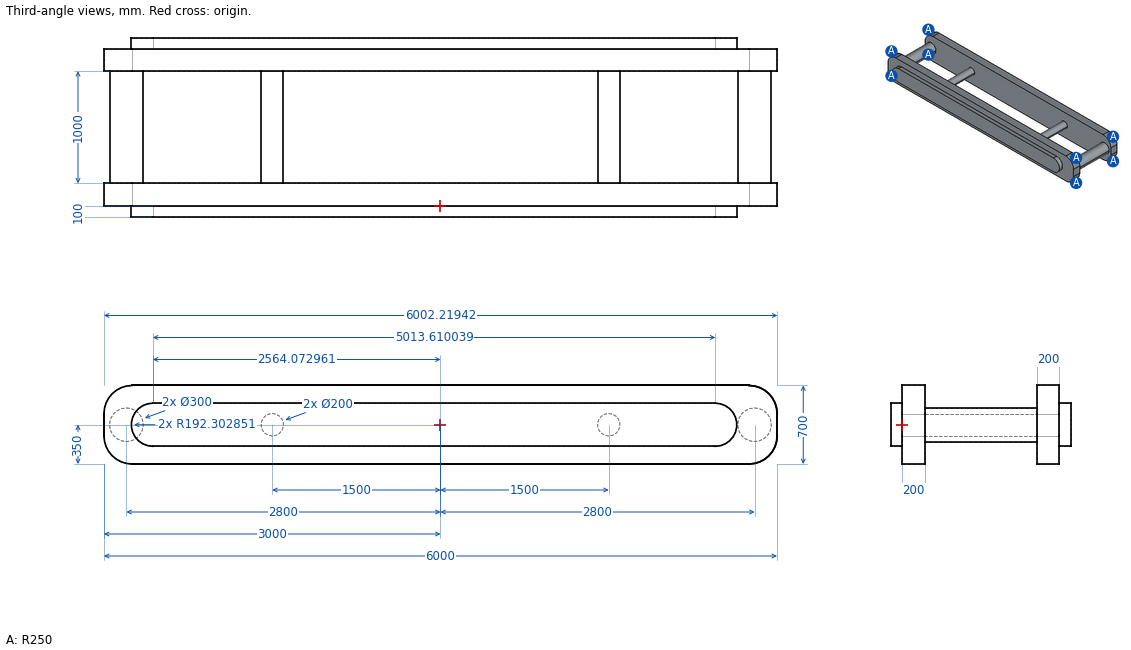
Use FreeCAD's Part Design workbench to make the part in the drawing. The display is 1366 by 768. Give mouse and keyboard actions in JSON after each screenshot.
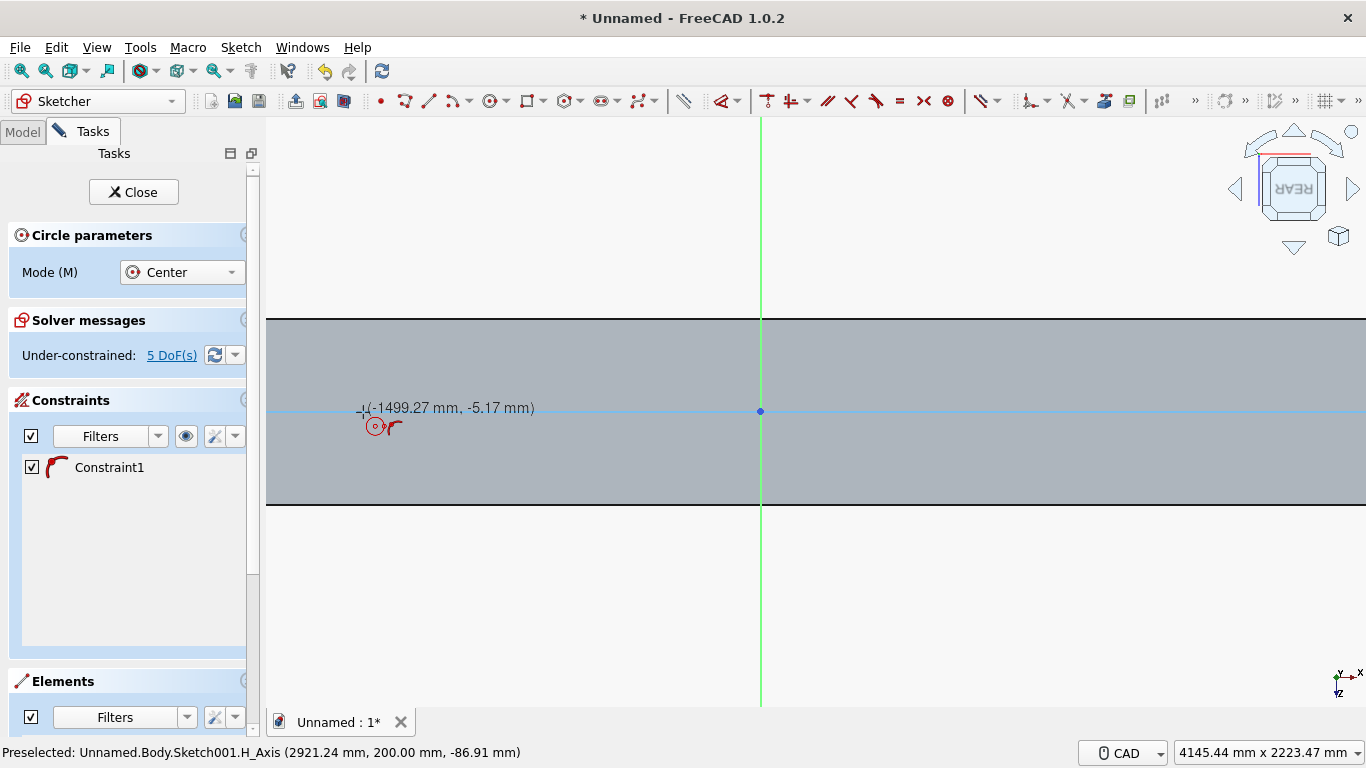
{"action": "left_click", "coordinate": [363, 412]}
{"action": "left_click", "coordinate": [382, 393]}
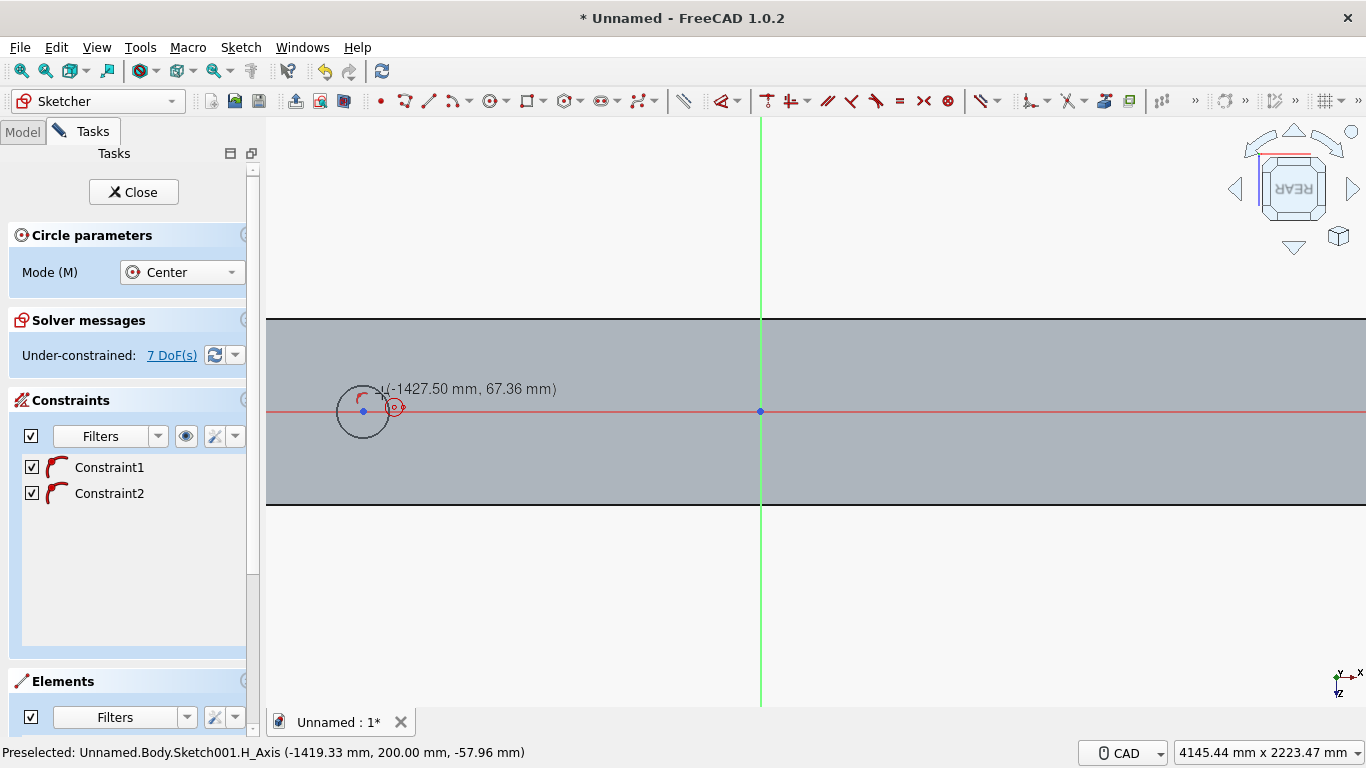
{"action": "left_click", "coordinate": [1159, 412]}
{"action": "left_click", "coordinate": [1178, 393]}
{"action": "key", "text": "Escape"}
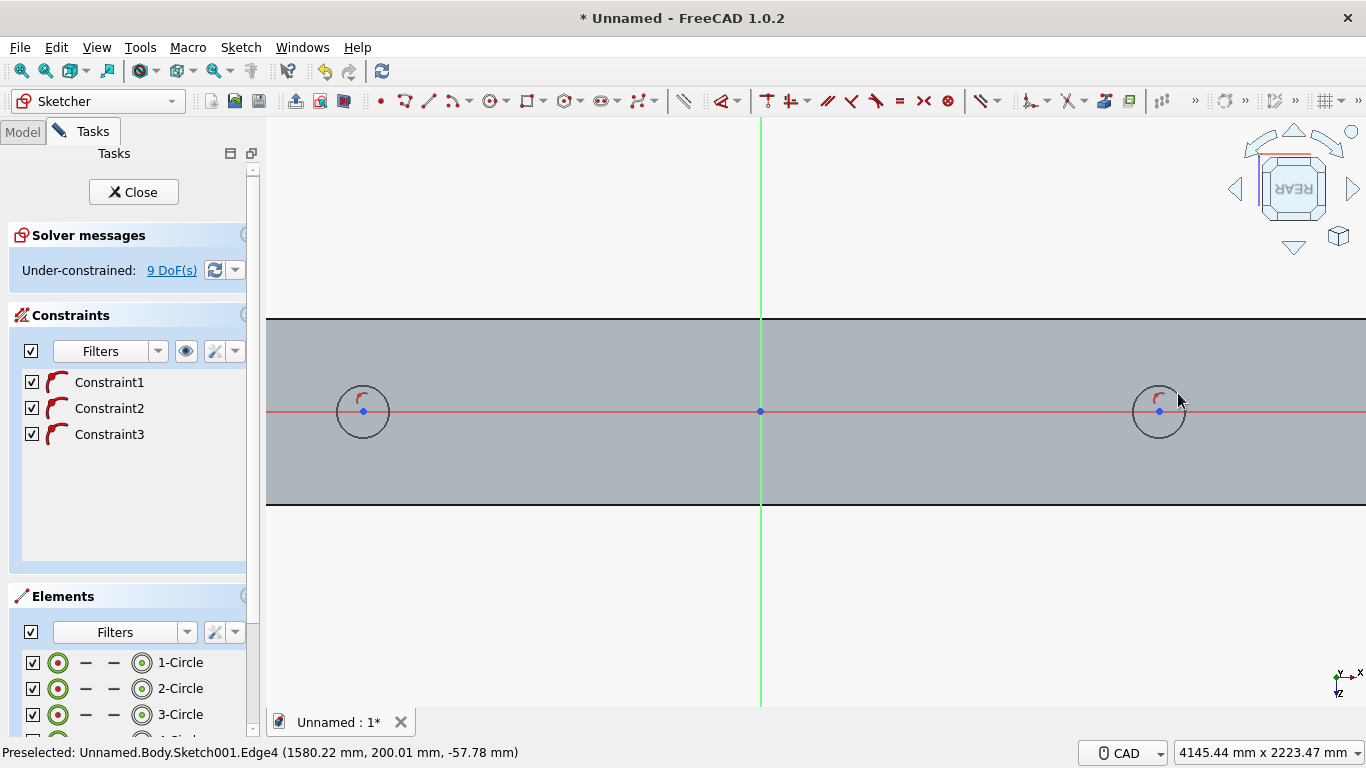
{"action": "scroll", "coordinate": [737, 412], "scroll_direction": "down", "scroll_amount": 4}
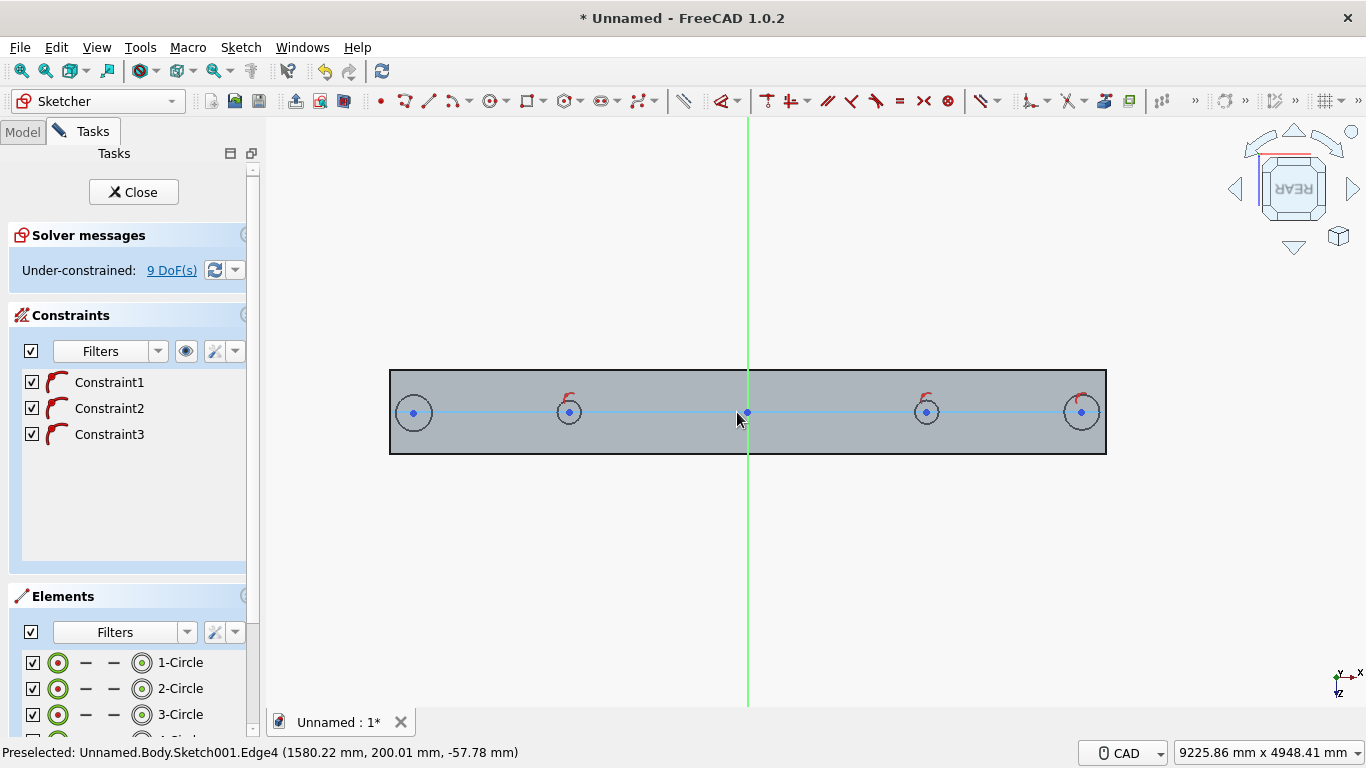
{"action": "left_click", "coordinate": [427, 400]}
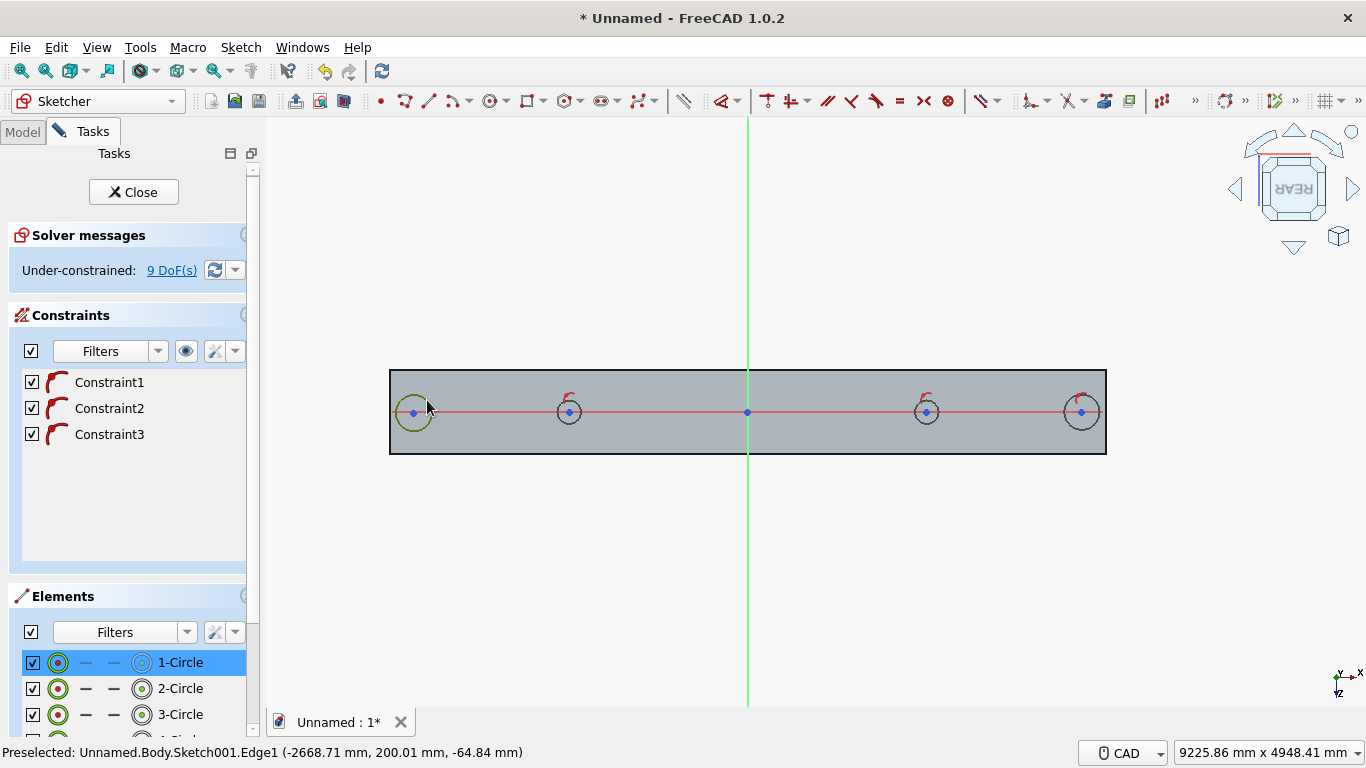
{"action": "left_click", "coordinate": [1094, 400]}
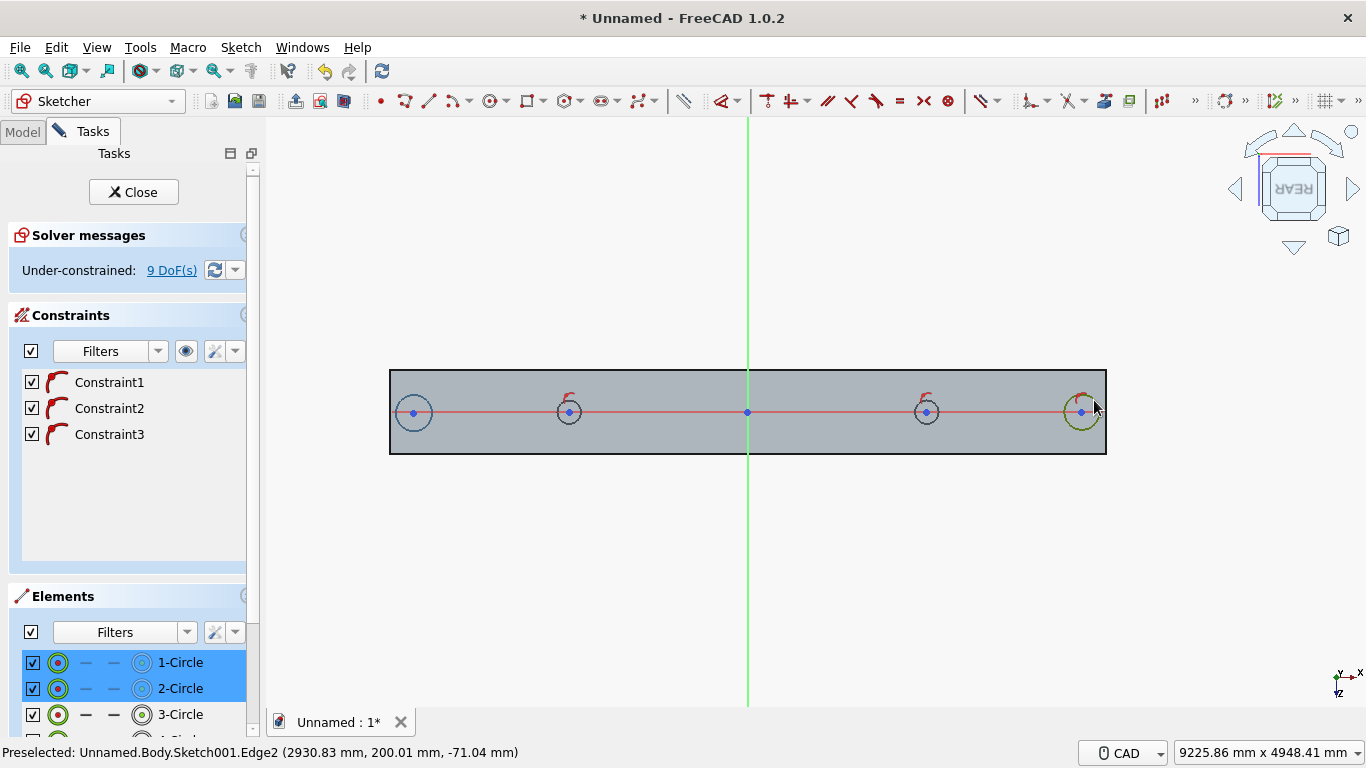
{"action": "left_click", "coordinate": [900, 102]}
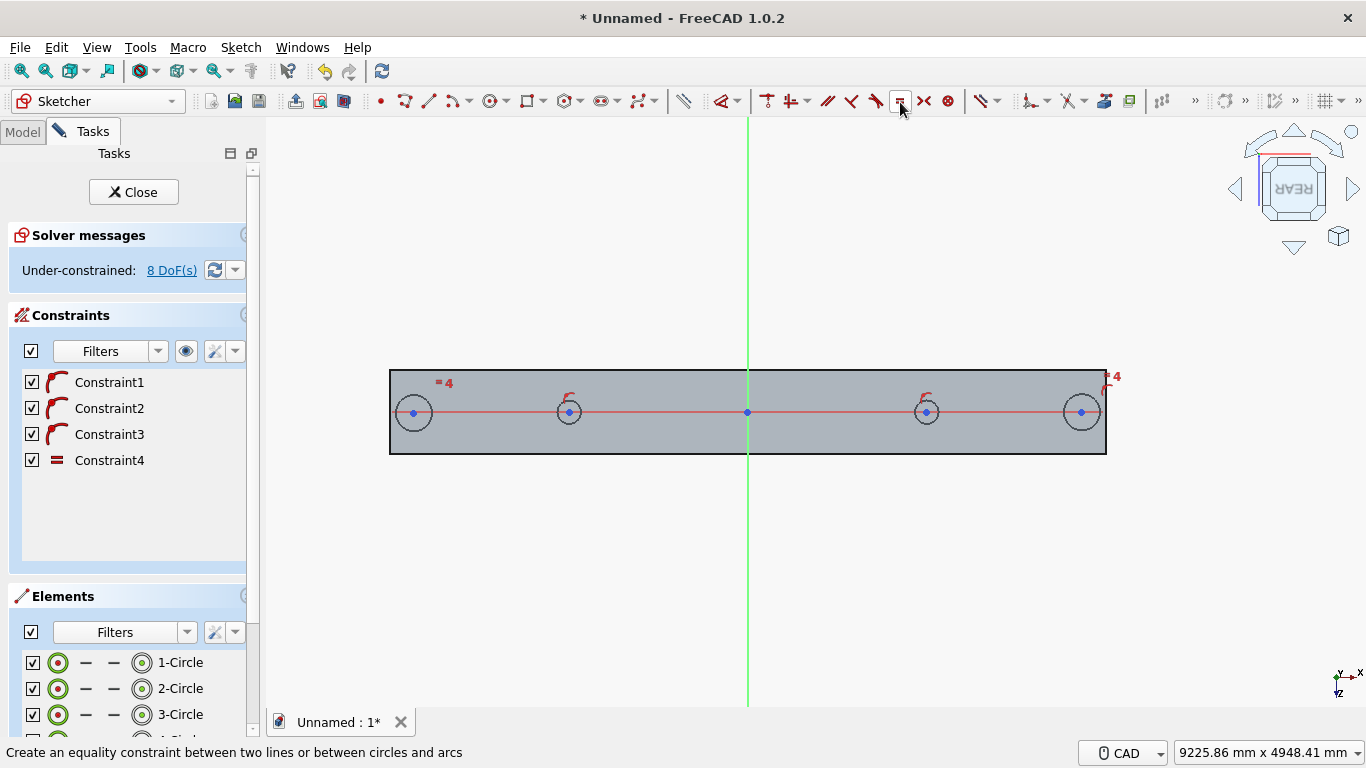
{"action": "left_click", "coordinate": [557, 412]}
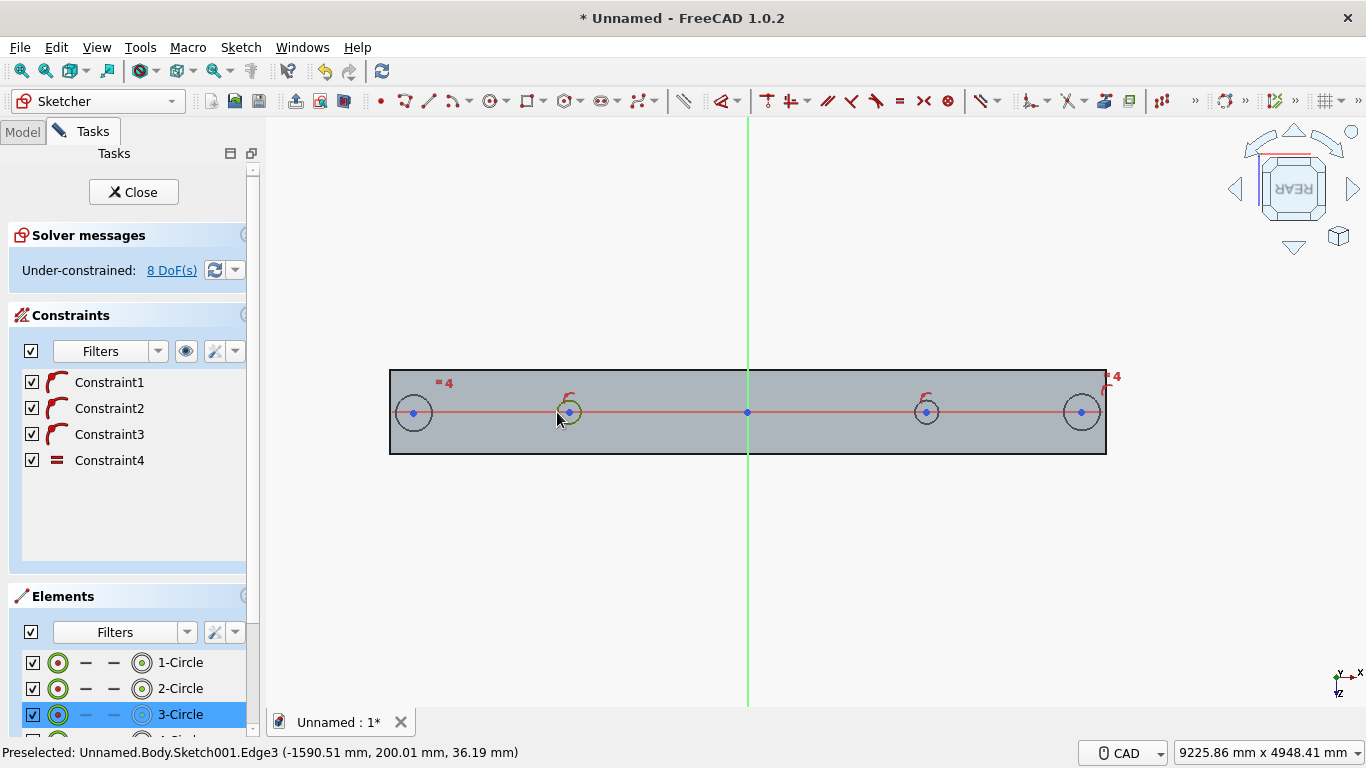
{"action": "left_click", "coordinate": [915, 412]}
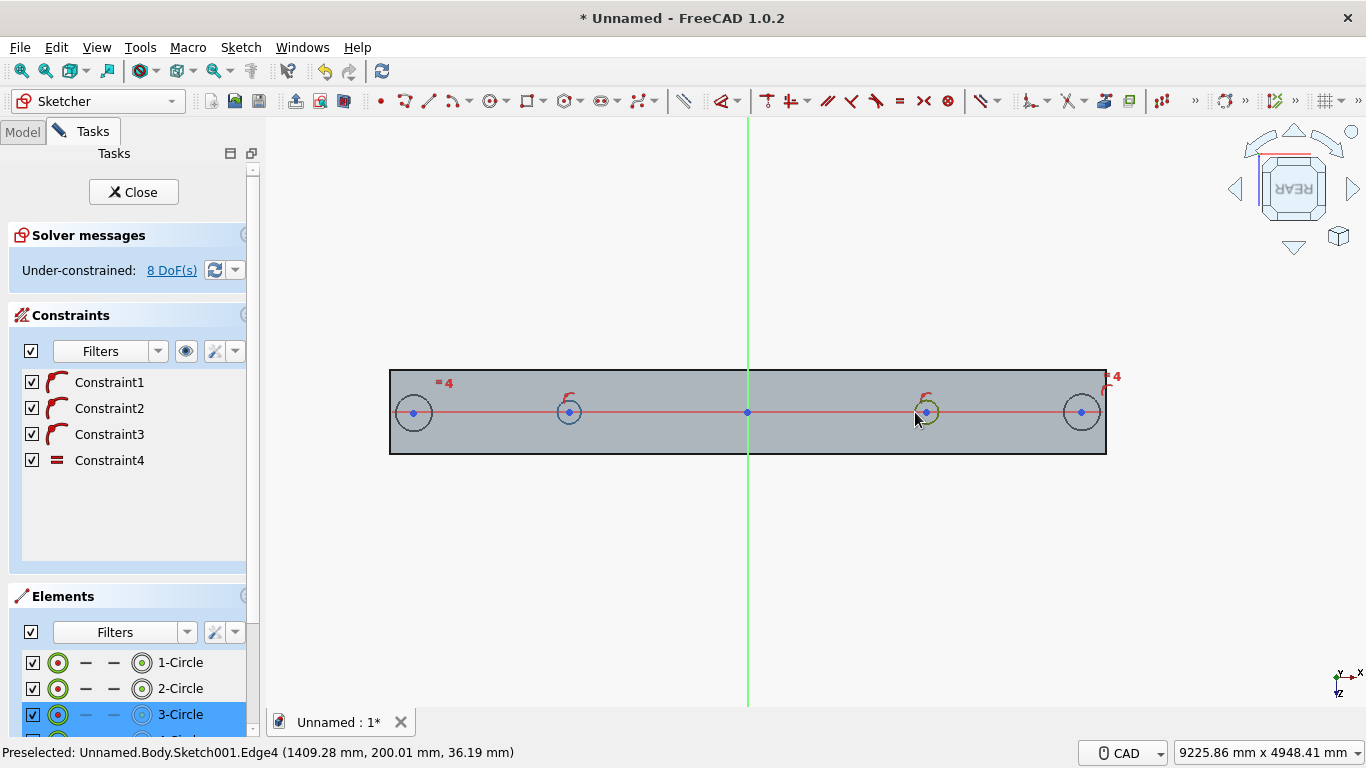
{"action": "left_click", "coordinate": [900, 102]}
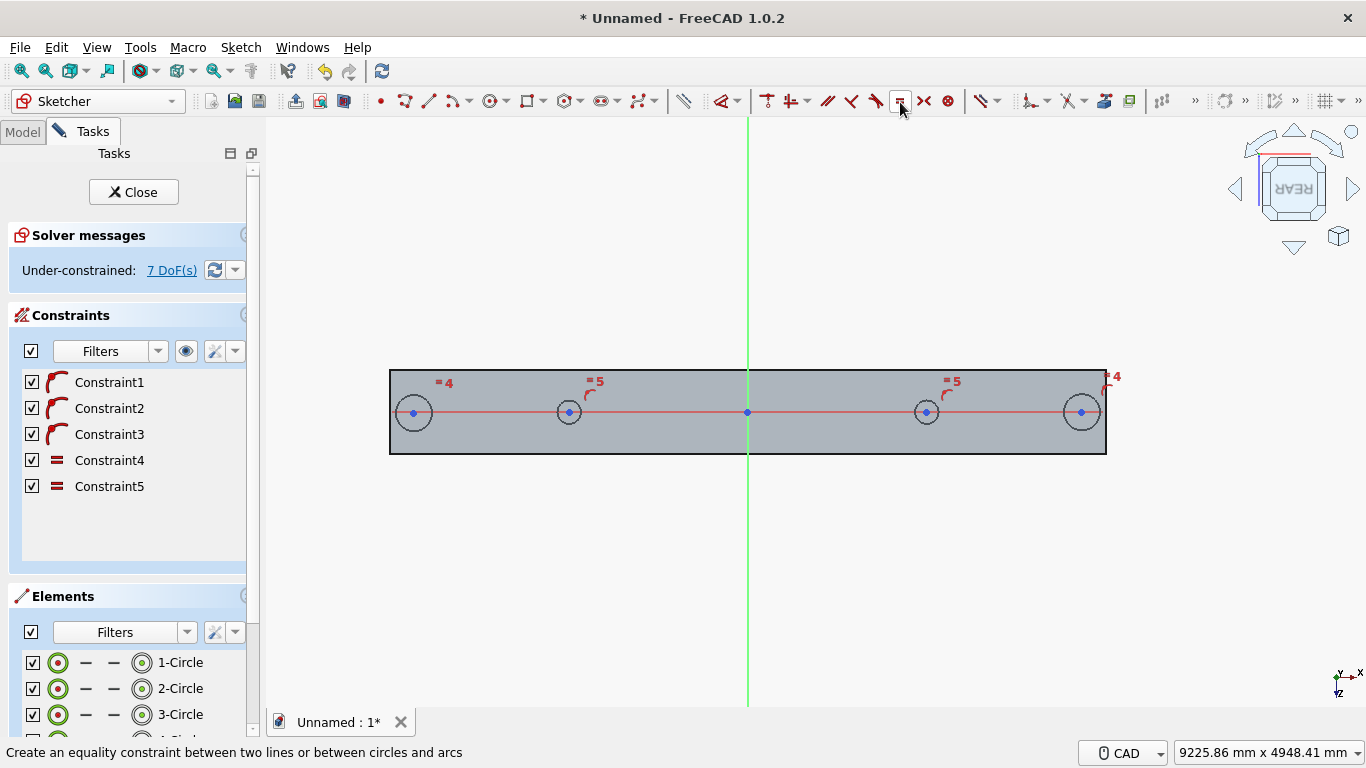
{"action": "left_click", "coordinate": [414, 413]}